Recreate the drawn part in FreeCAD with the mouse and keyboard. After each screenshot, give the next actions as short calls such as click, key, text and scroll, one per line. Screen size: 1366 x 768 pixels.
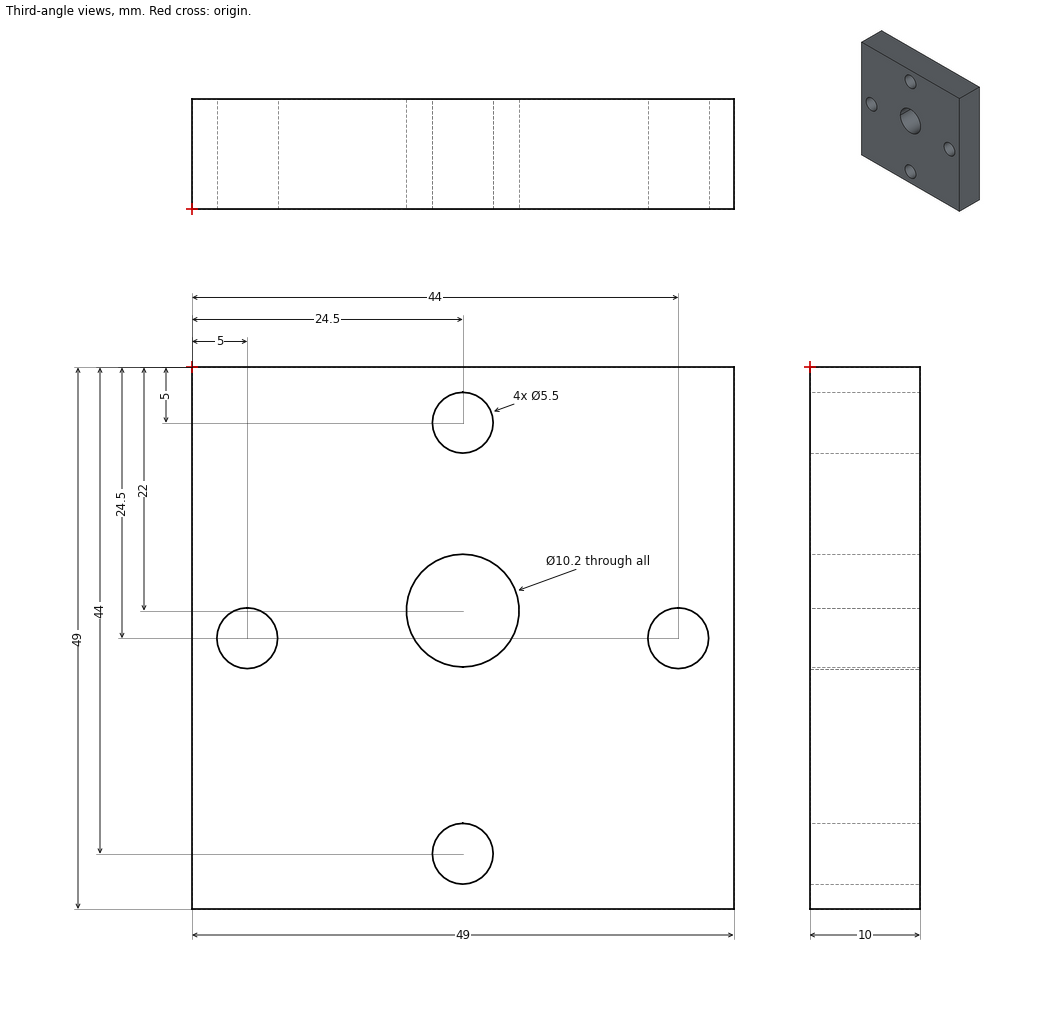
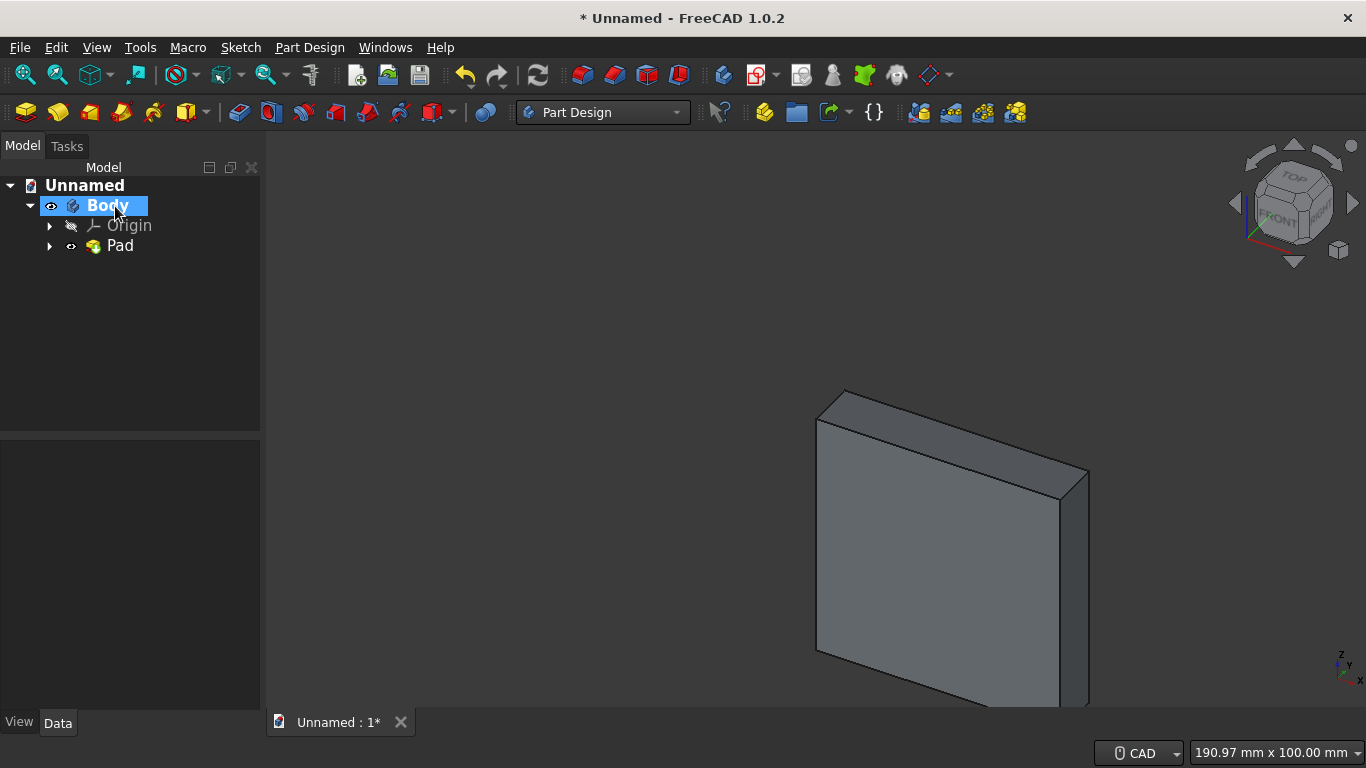
click(26, 76)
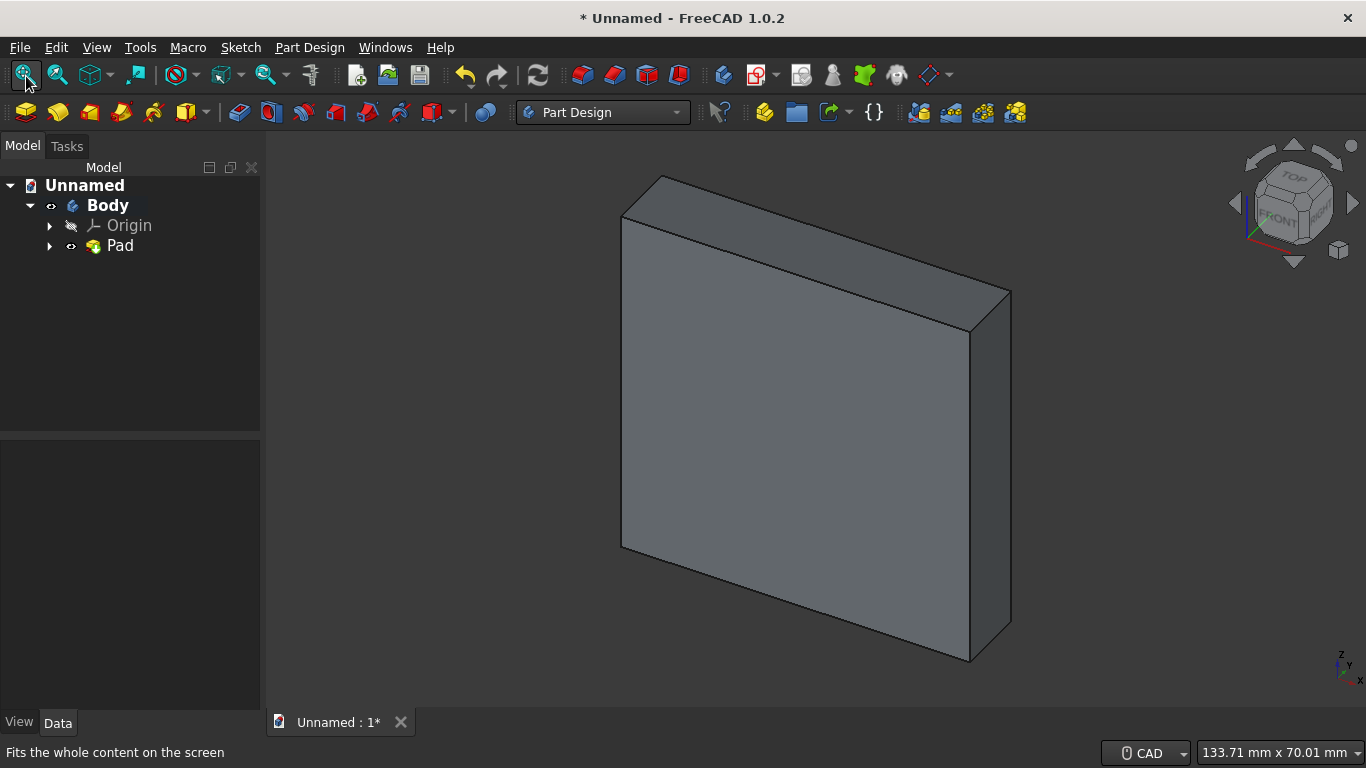
key(4)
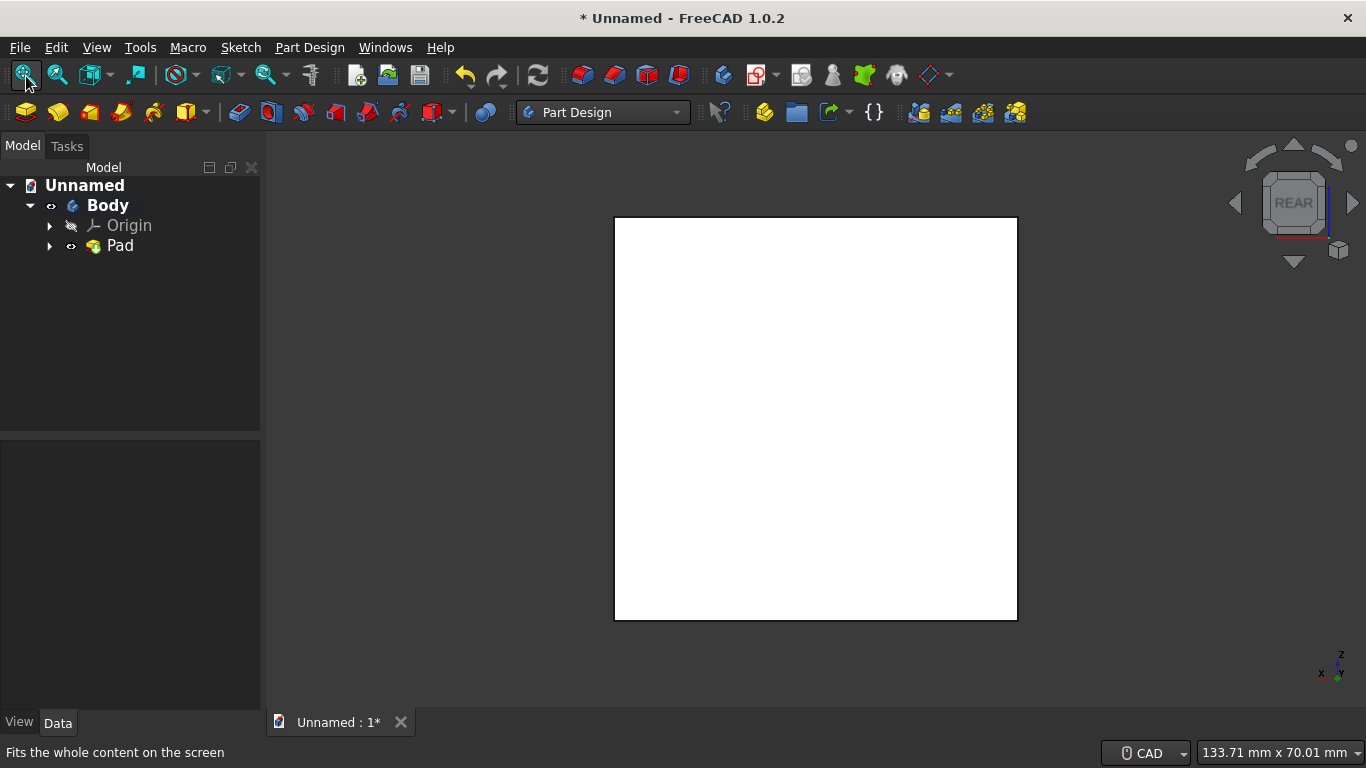
click(816, 418)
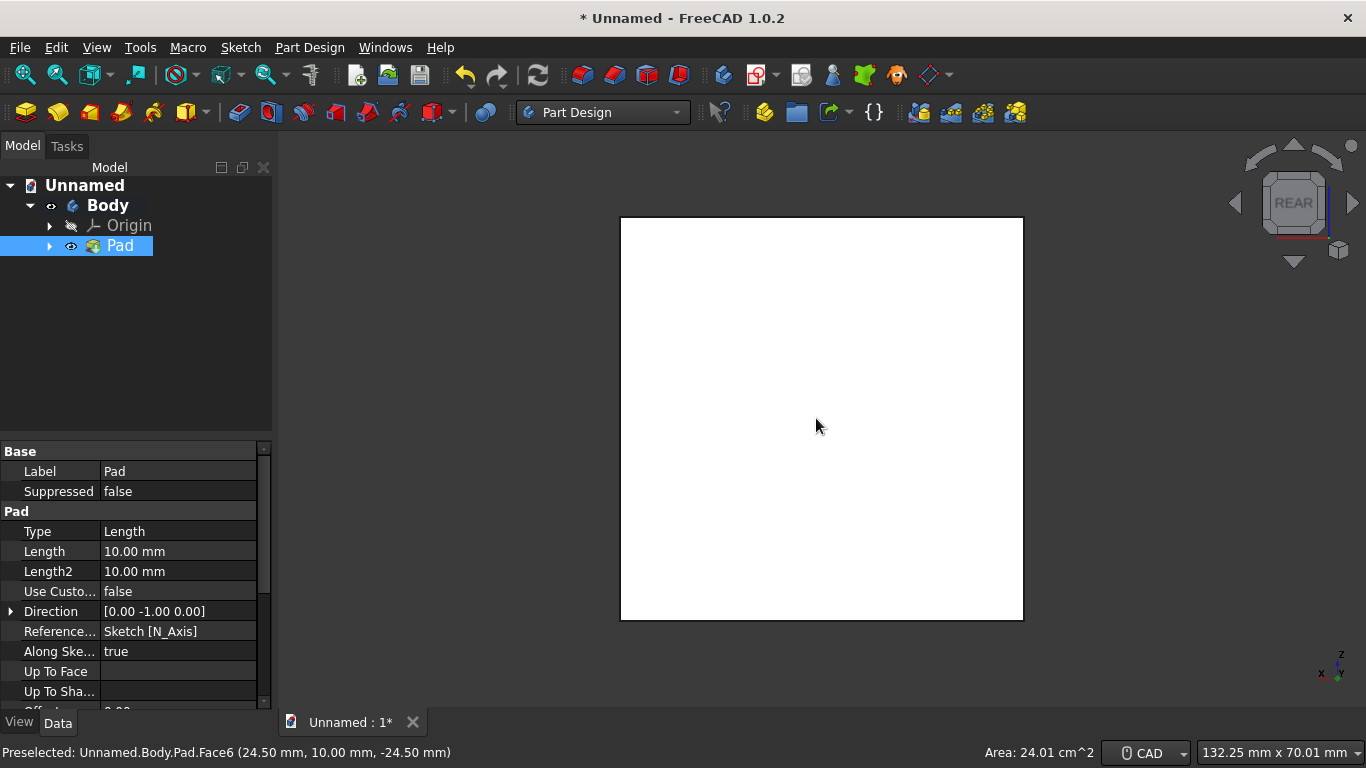
click(756, 76)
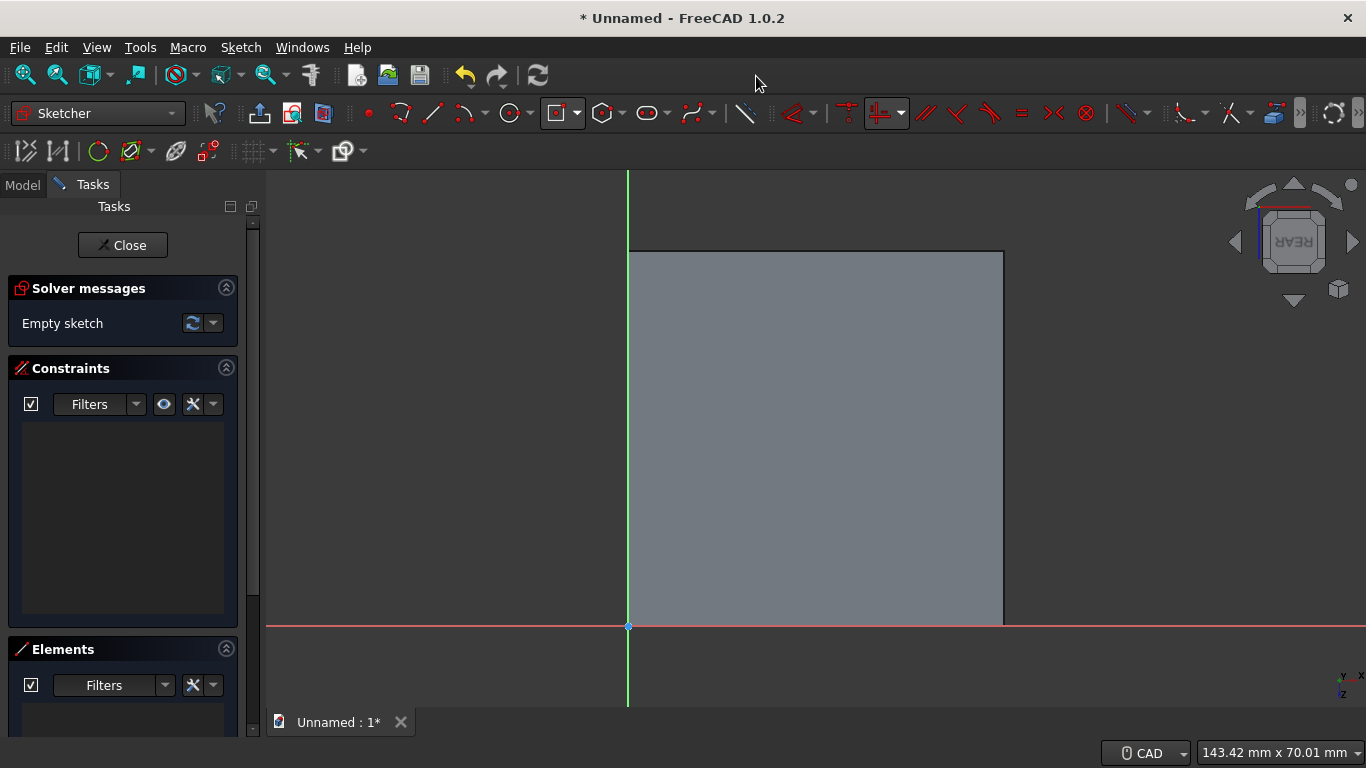
click(510, 114)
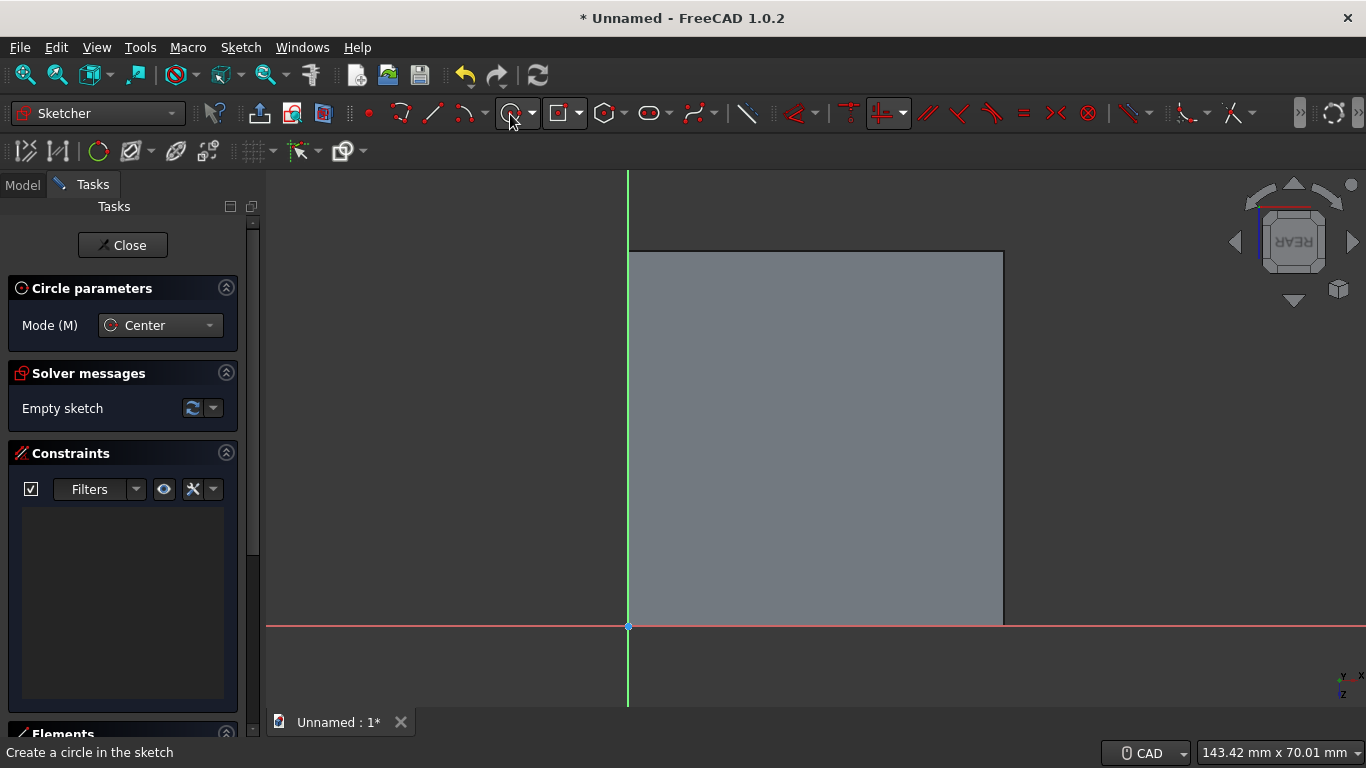
click(816, 588)
click(831, 573)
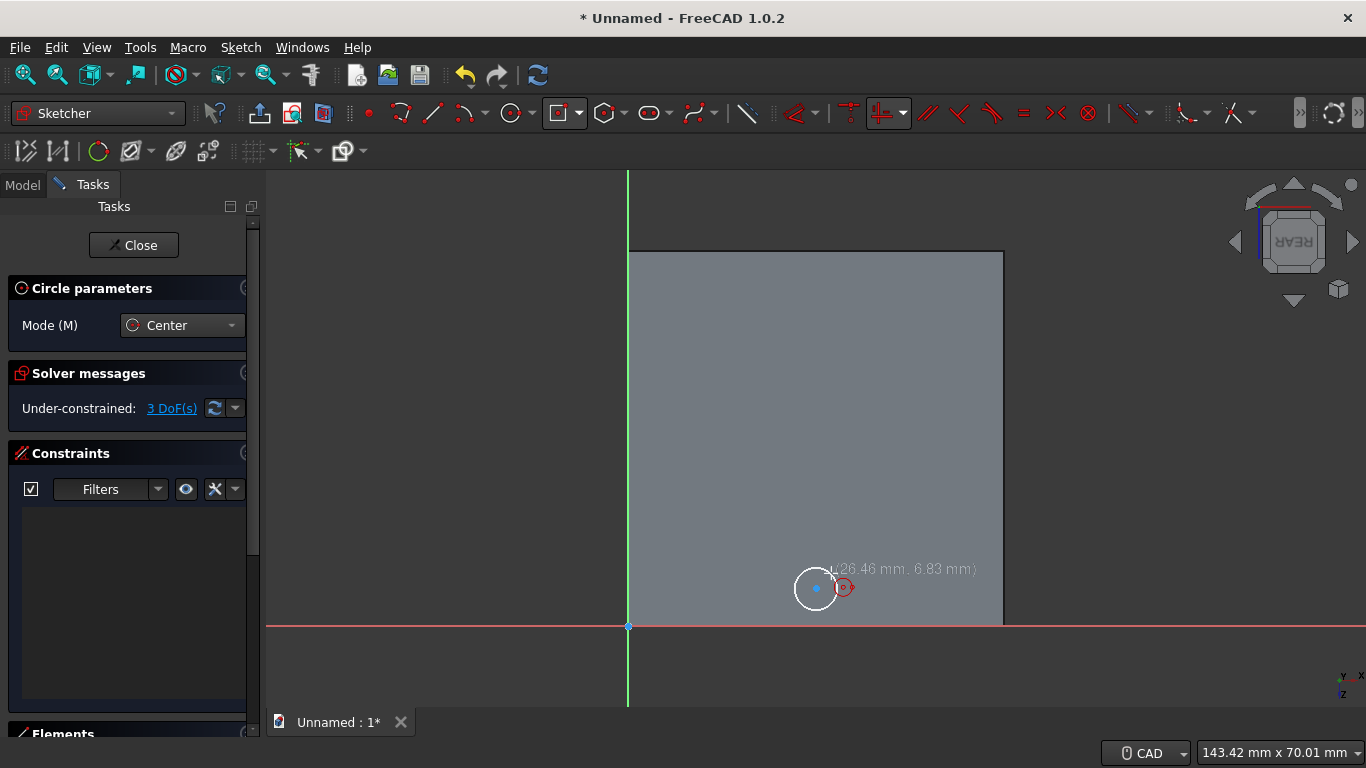
click(966, 439)
click(980, 424)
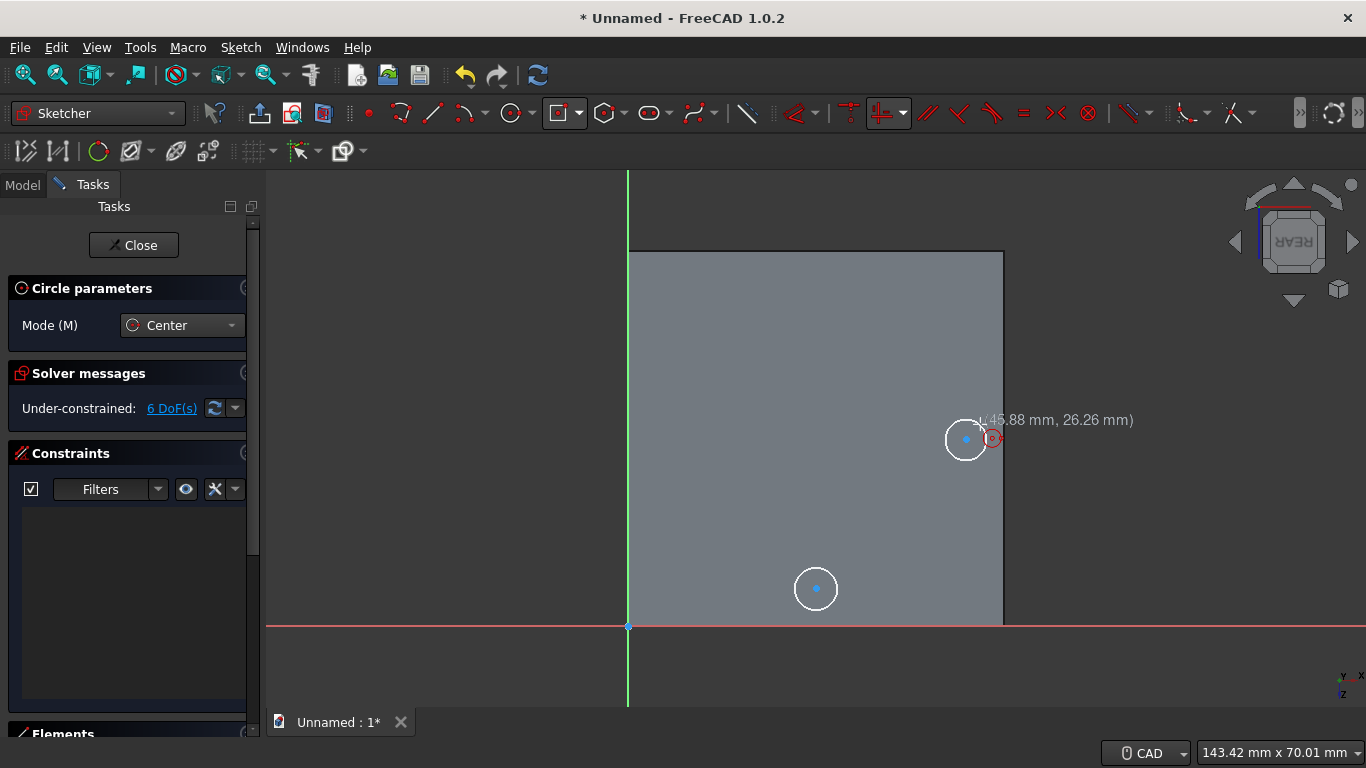
click(816, 289)
click(831, 274)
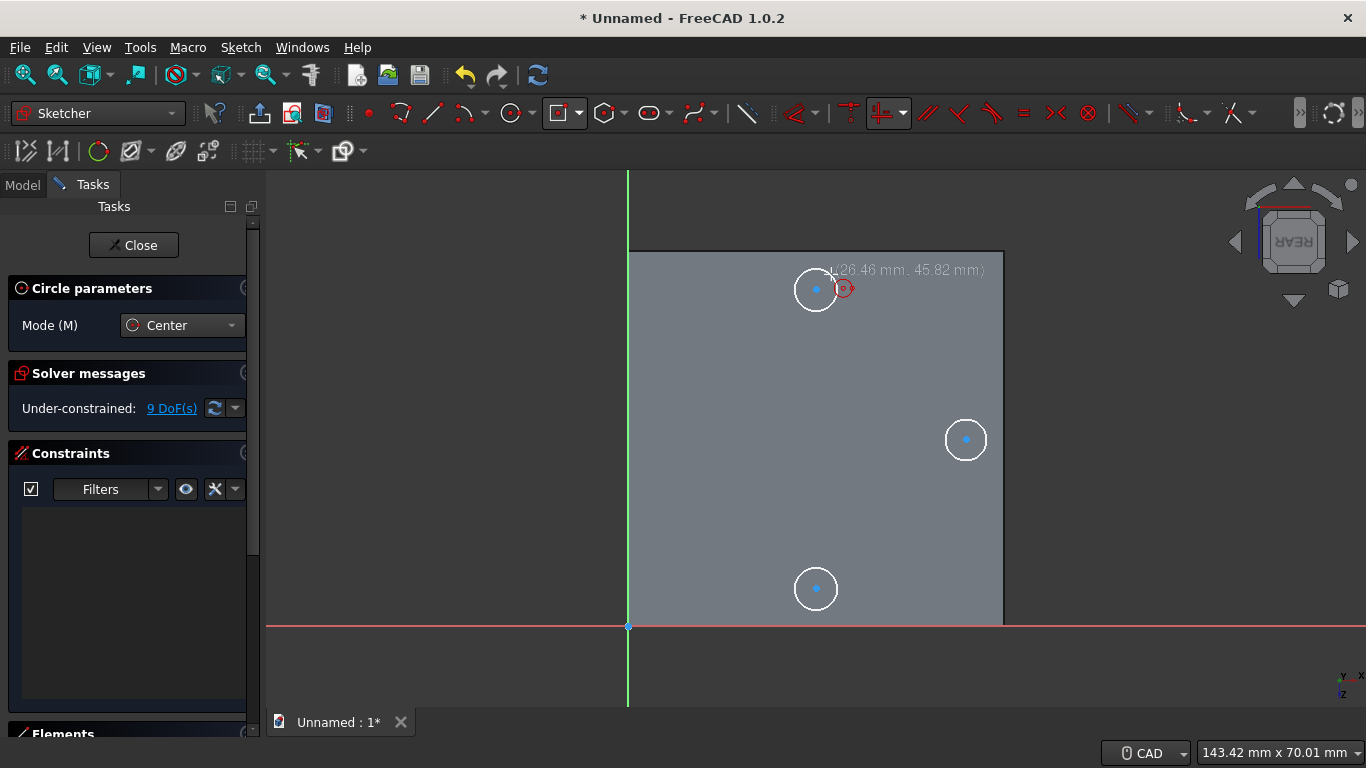
click(666, 439)
click(681, 424)
key(Escape)